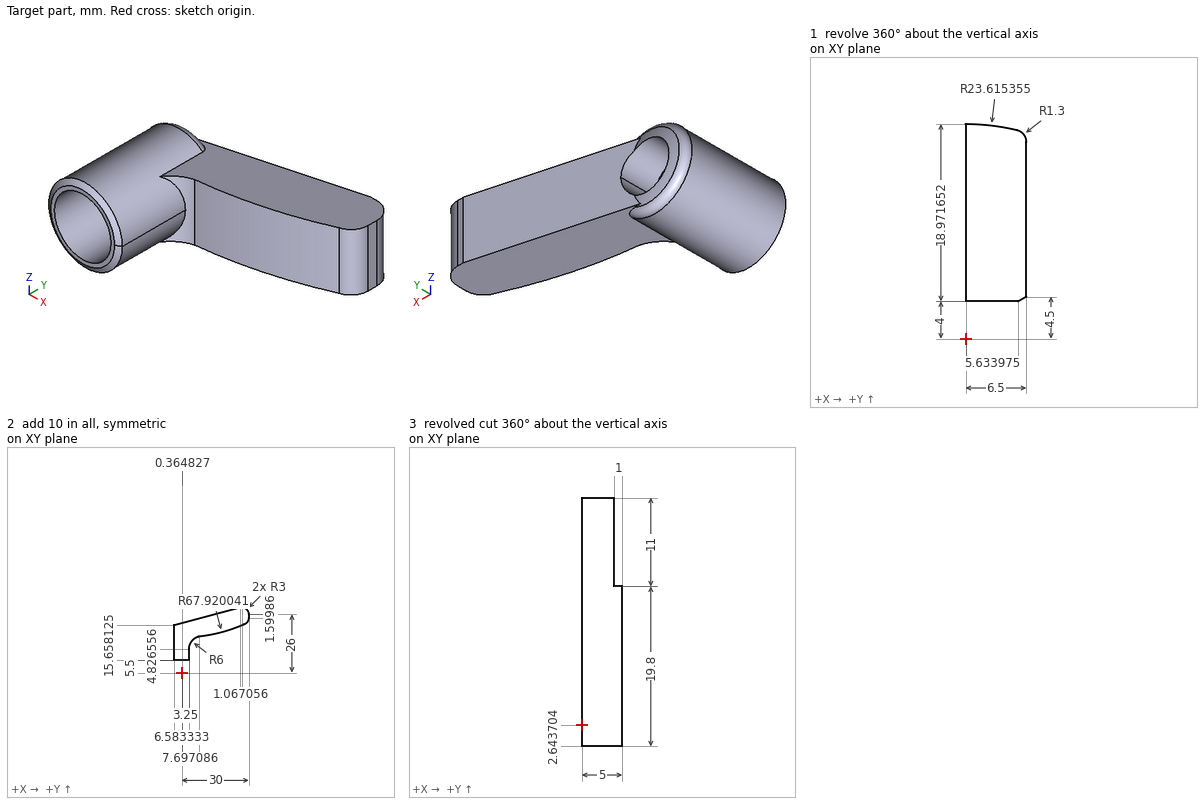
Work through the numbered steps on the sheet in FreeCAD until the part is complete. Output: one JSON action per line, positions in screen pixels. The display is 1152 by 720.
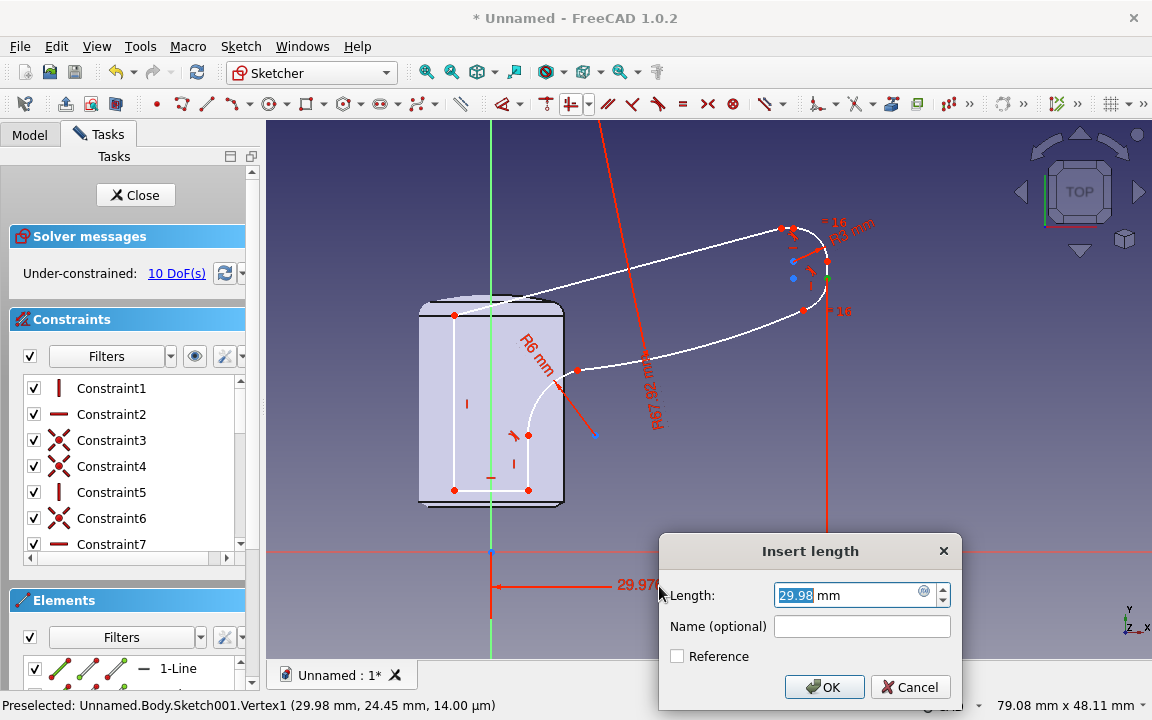
{"action": "type", "text": "30"}
{"action": "key", "text": "Return"}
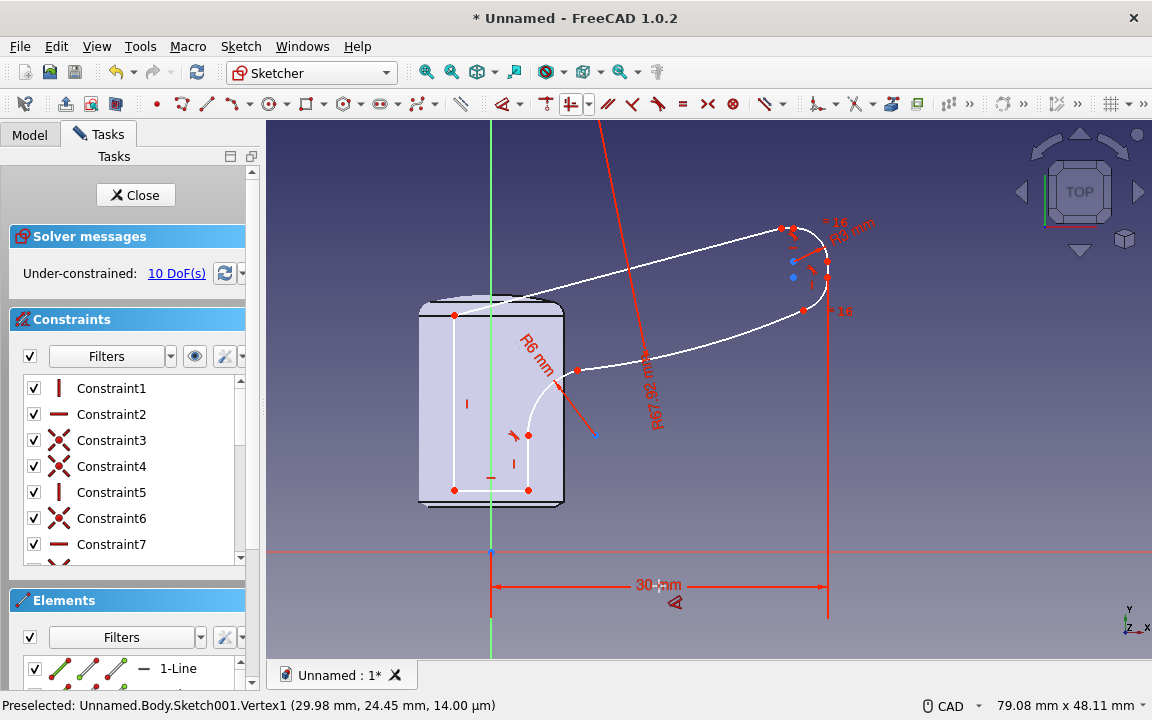
{"action": "left_click", "coordinate": [828, 262]}
{"action": "left_click", "coordinate": [862, 407]}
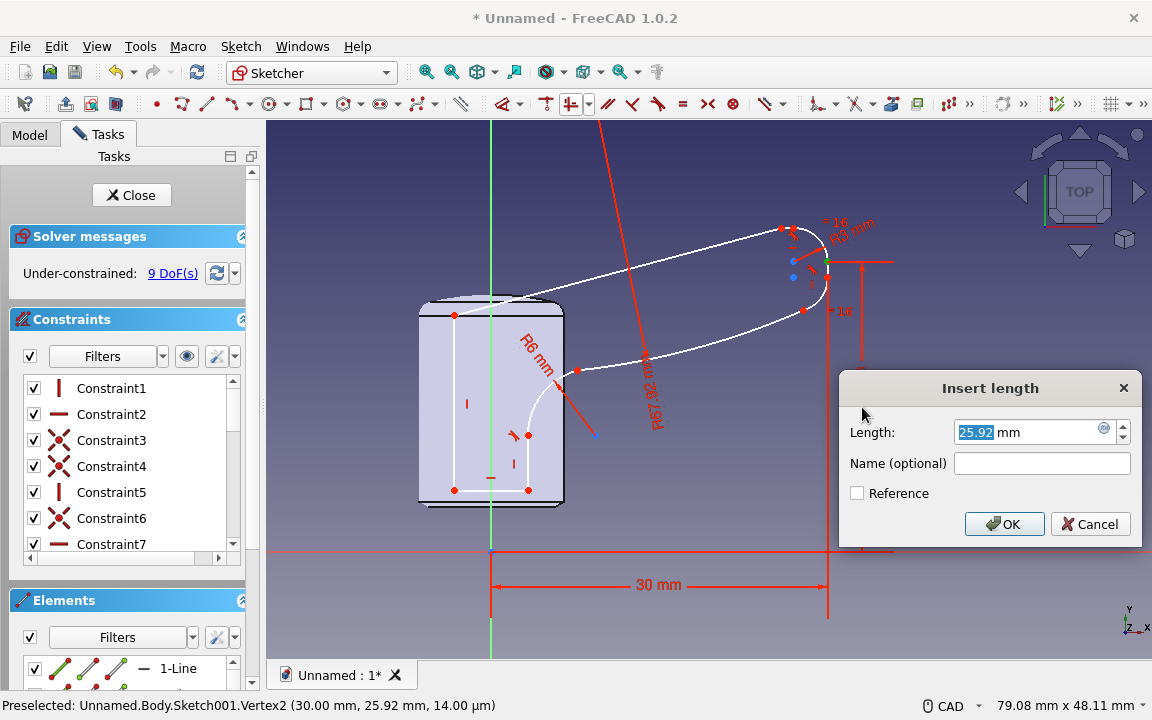
{"action": "type", "text": "26"}
{"action": "key", "text": "Return"}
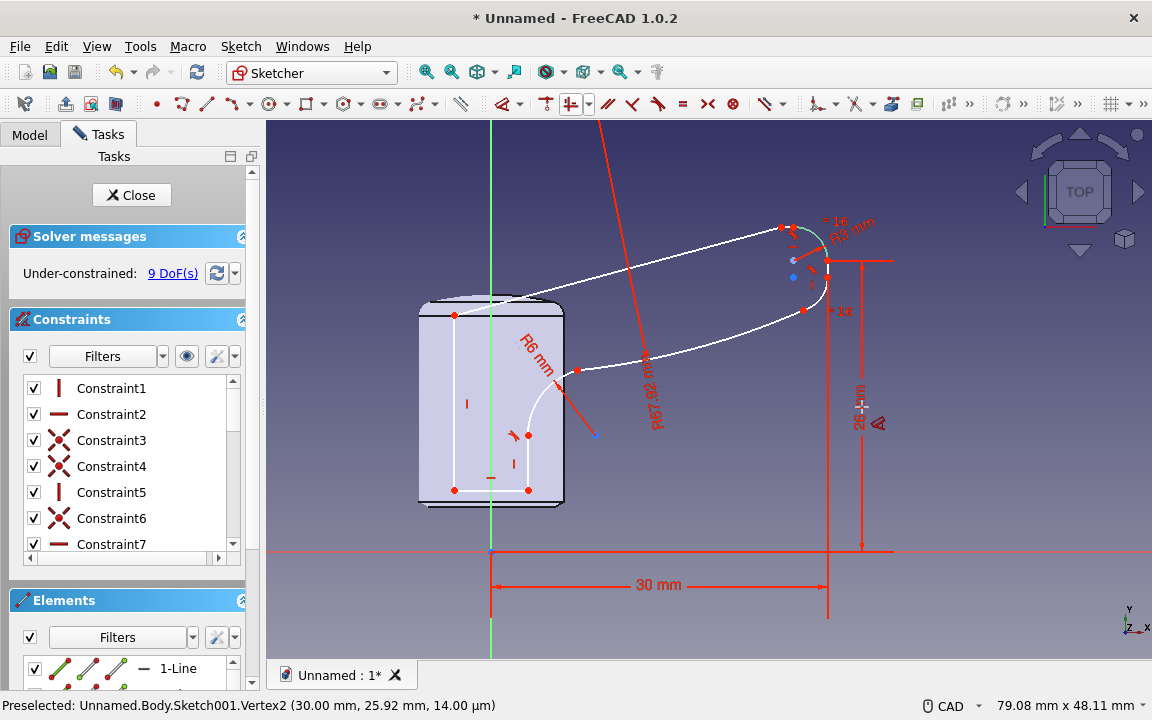
{"action": "left_click", "coordinate": [454, 491]}
{"action": "left_click", "coordinate": [420, 521]}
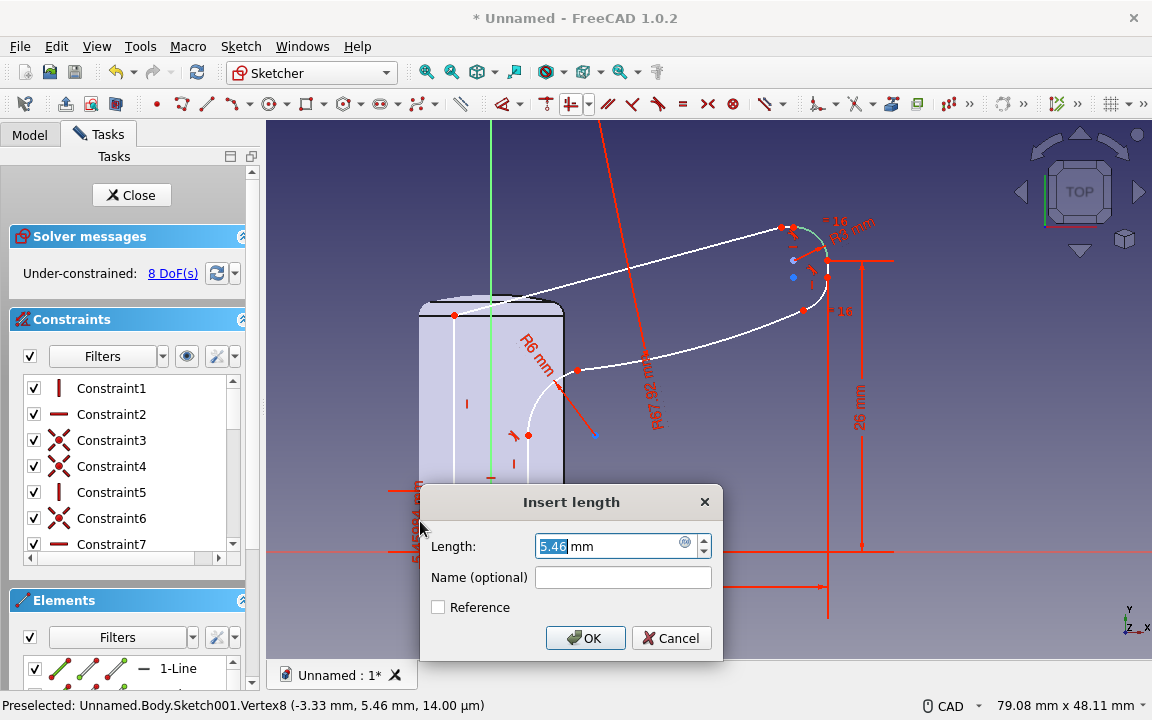
{"action": "type", "text": "5.5"}
{"action": "key", "text": "Return"}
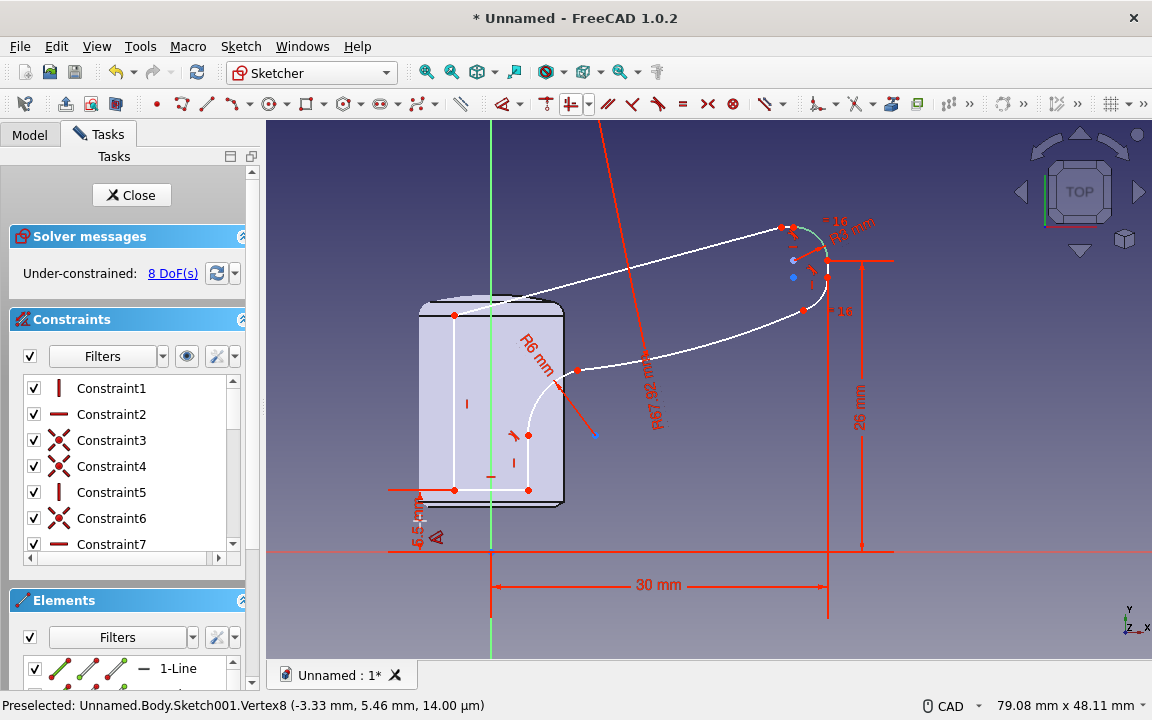
{"action": "left_click", "coordinate": [528, 490]}
{"action": "left_click", "coordinate": [510, 586]}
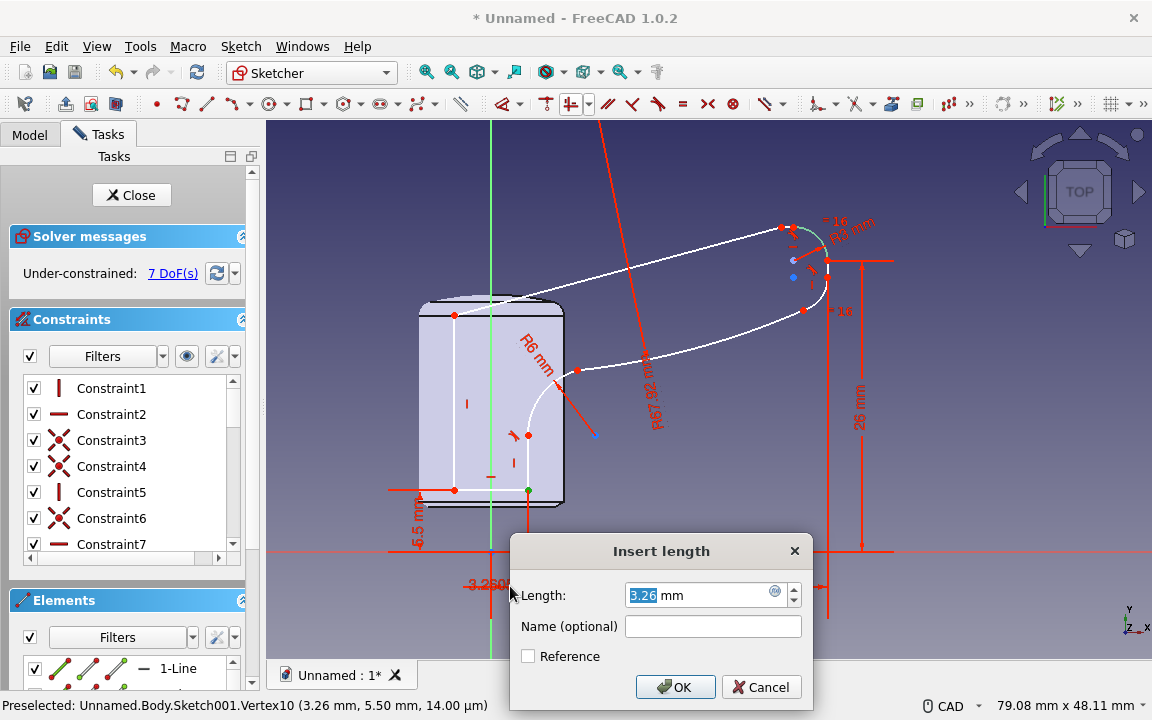
{"action": "type", "text": "3.25"}
{"action": "key", "text": "Return"}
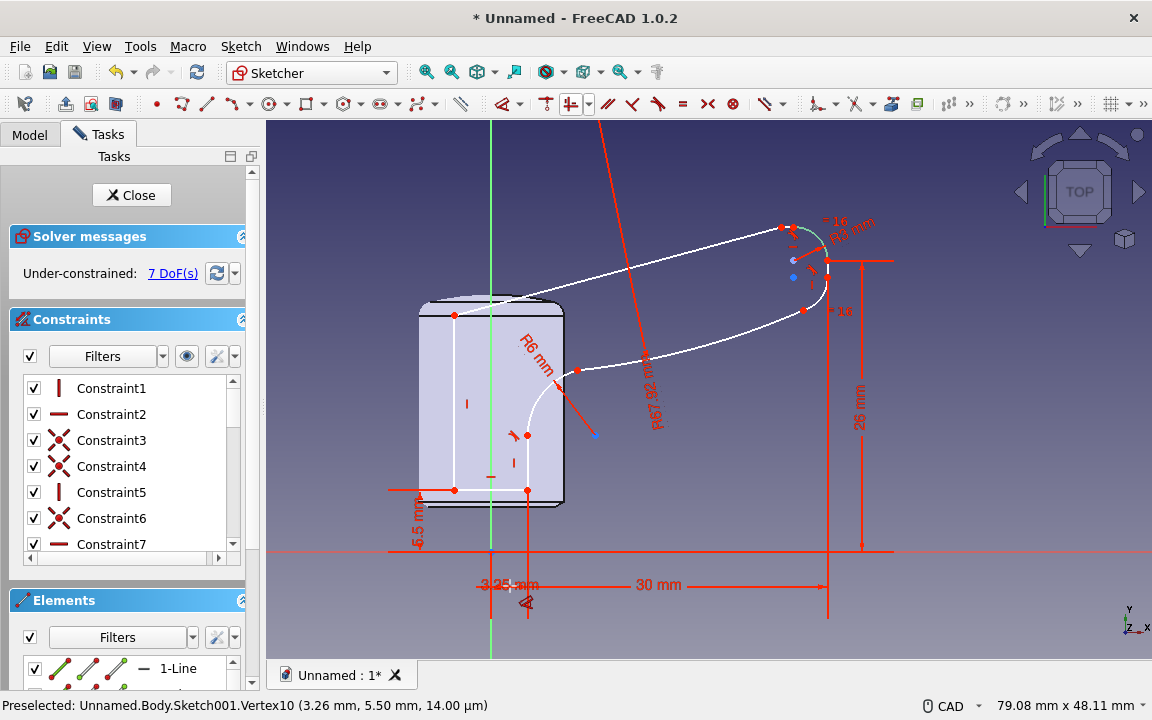
{"action": "scroll", "coordinate": [828, 269], "scroll_direction": "up", "scroll_amount": 4}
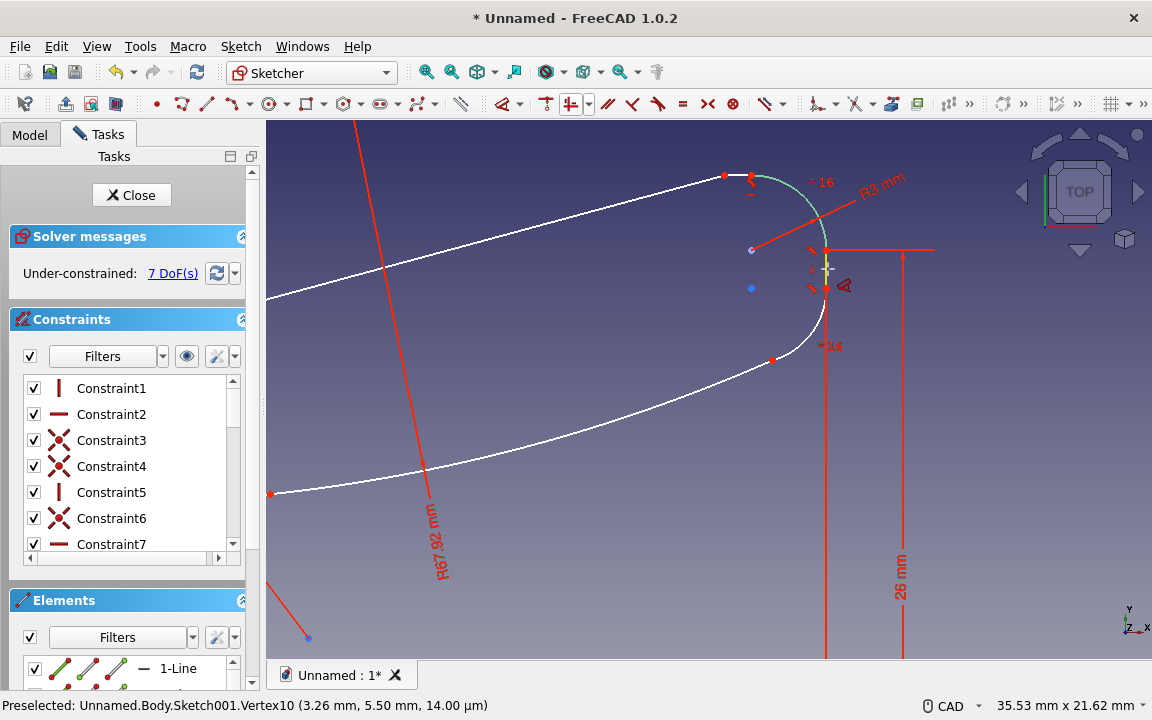
{"action": "left_click", "coordinate": [826, 269]}
{"action": "left_click", "coordinate": [860, 269]}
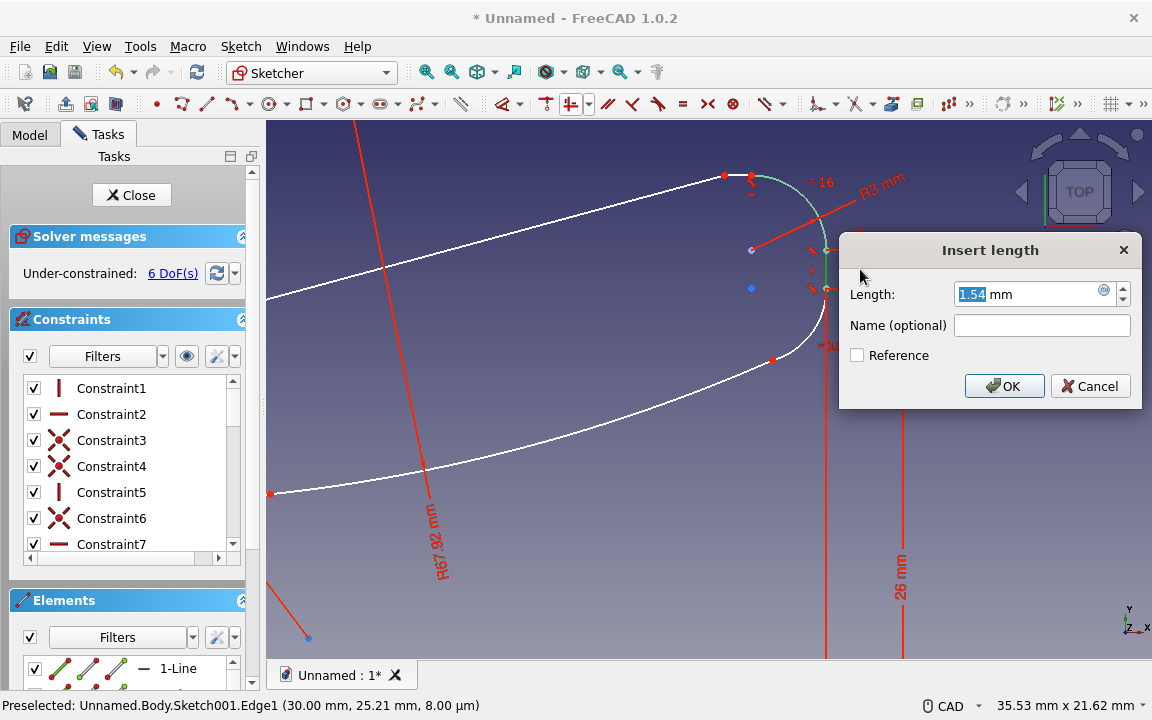
{"action": "type", "text": "1.59986"}
{"action": "key", "text": "Return"}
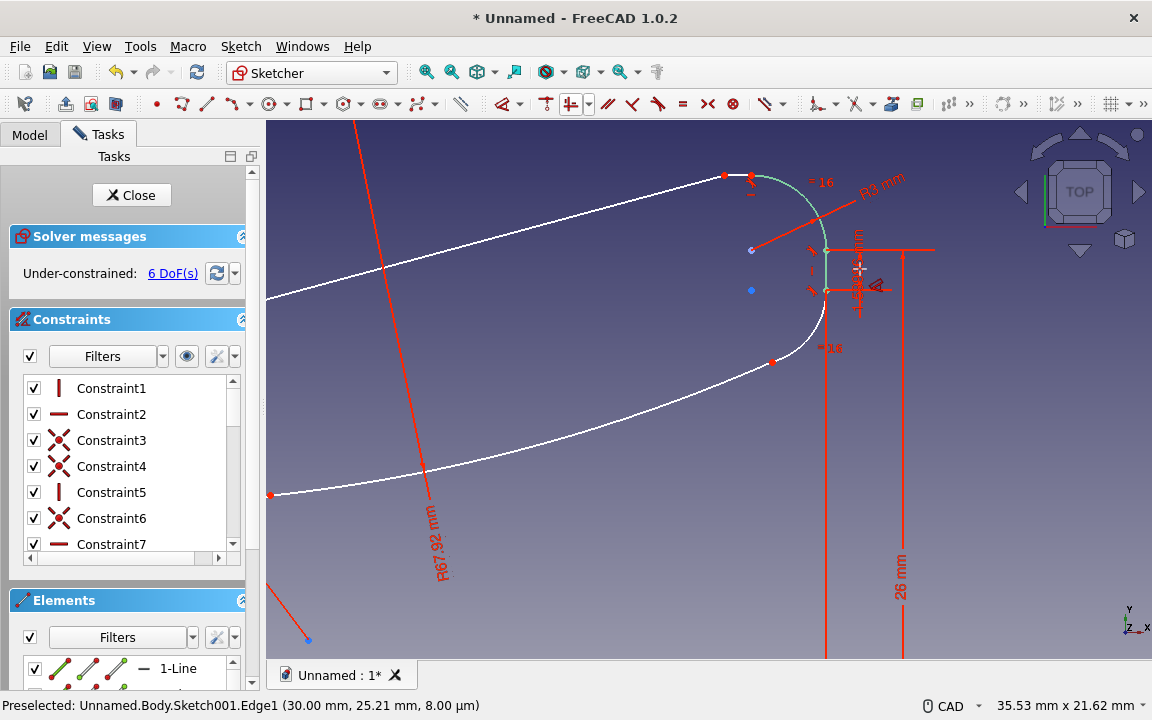
{"action": "scroll", "coordinate": [741, 175], "scroll_direction": "up", "scroll_amount": 3}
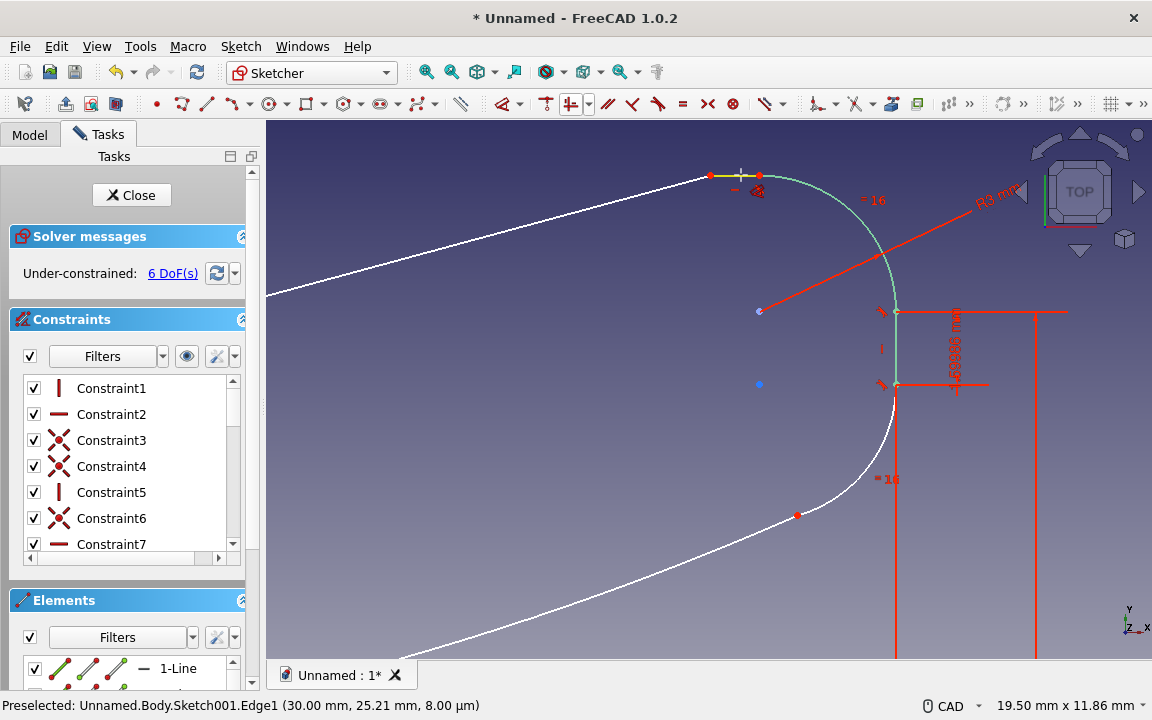
{"action": "left_click", "coordinate": [740, 176]}
{"action": "left_click", "coordinate": [735, 210]}